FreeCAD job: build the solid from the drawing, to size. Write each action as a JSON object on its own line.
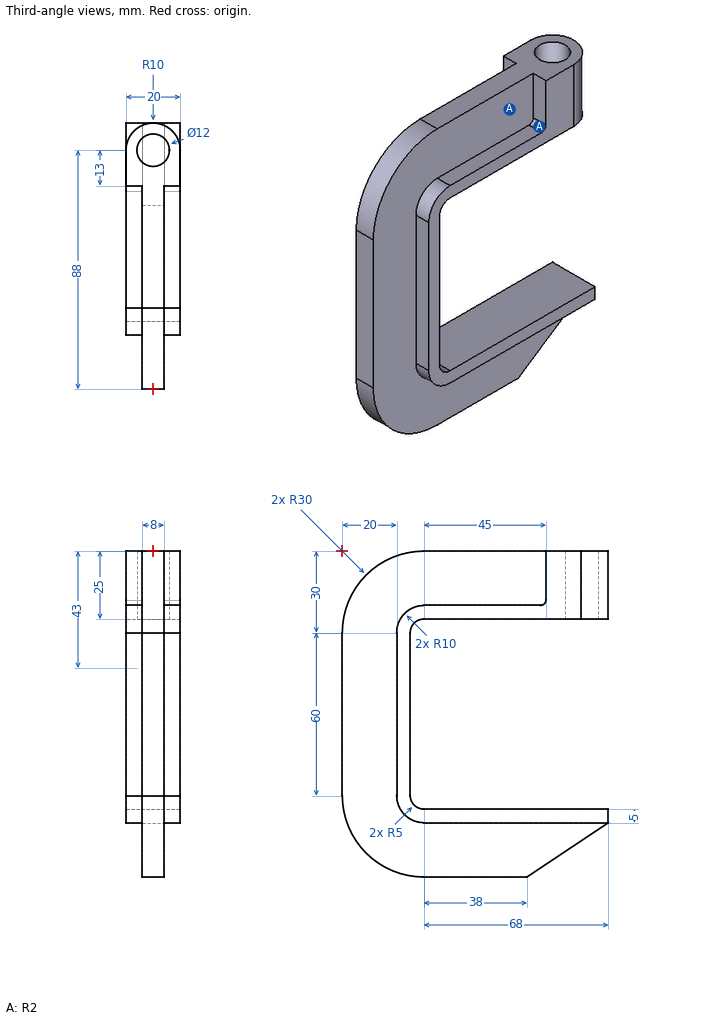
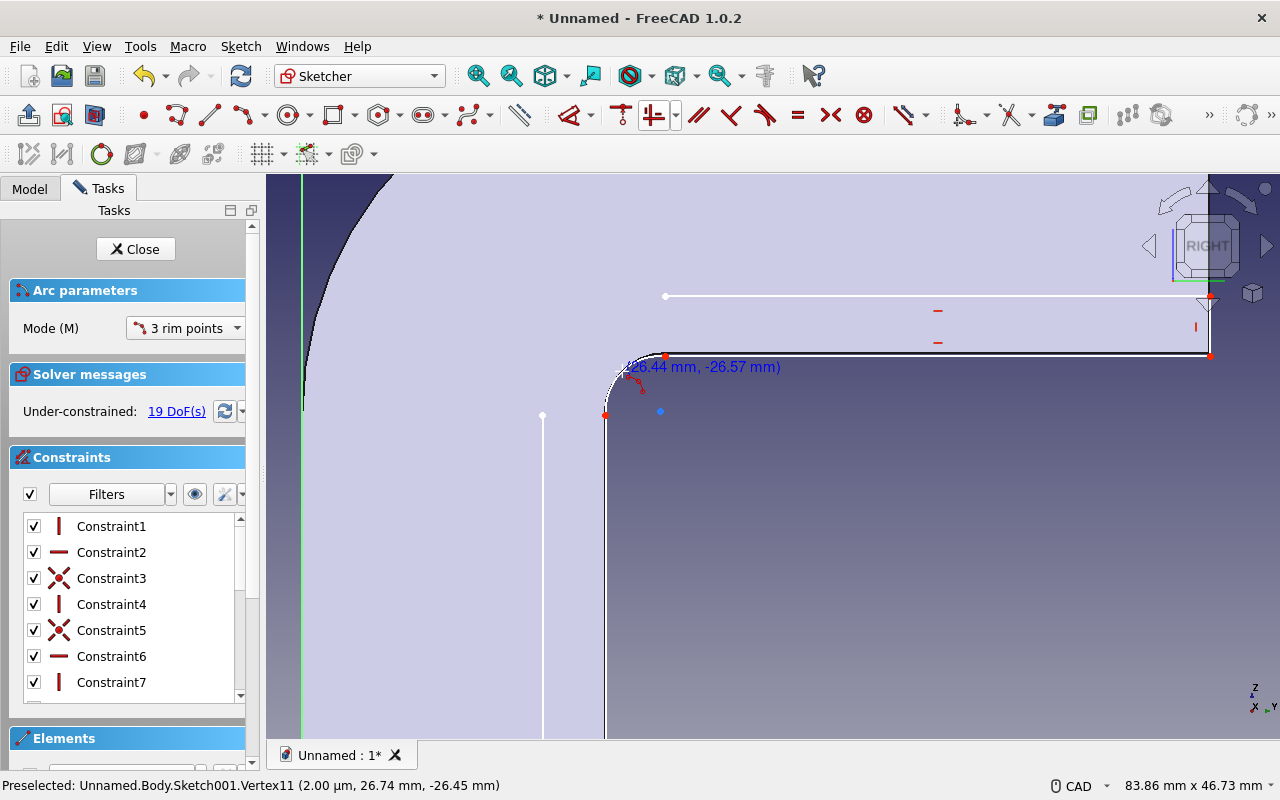
{"action": "left_click", "coordinate": [666, 296]}
{"action": "left_click", "coordinate": [543, 416]}
{"action": "left_click", "coordinate": [580, 328]}
{"action": "key", "text": "Escape"}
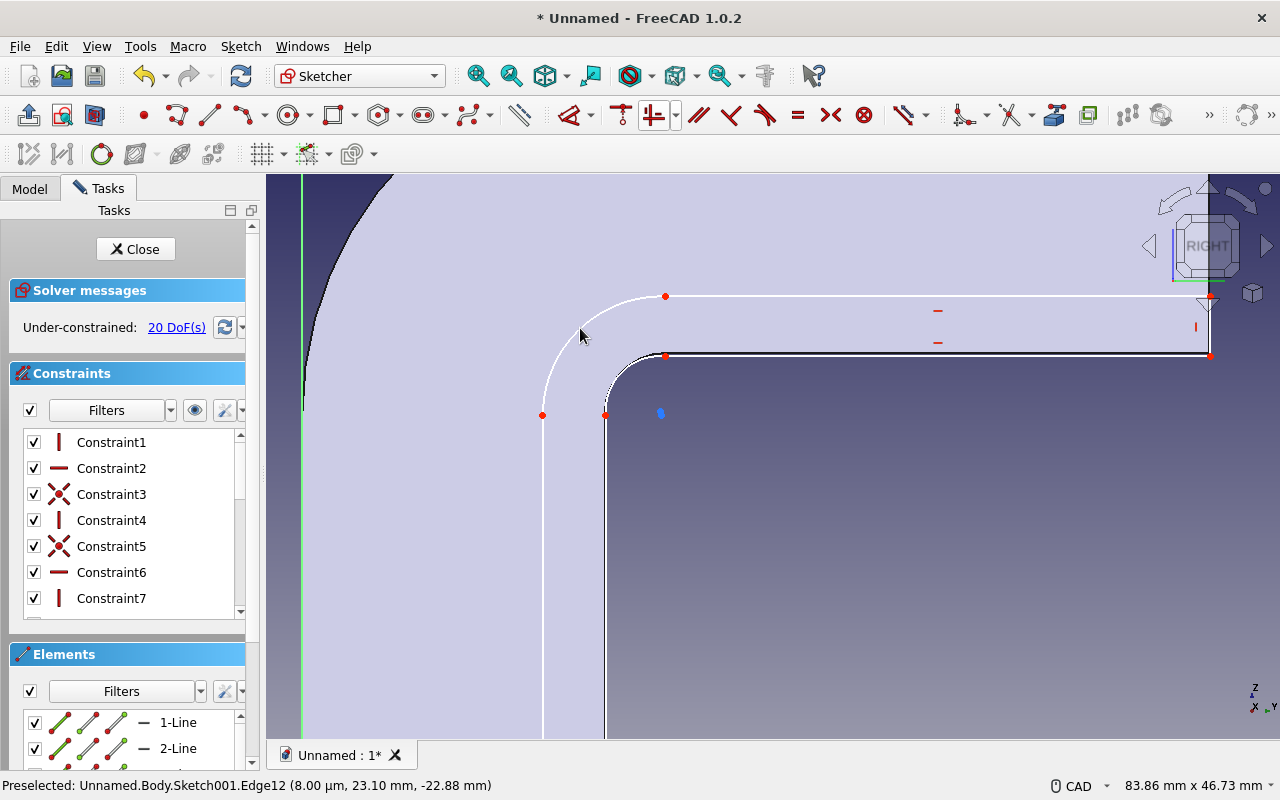
{"action": "left_click", "coordinate": [543, 634]}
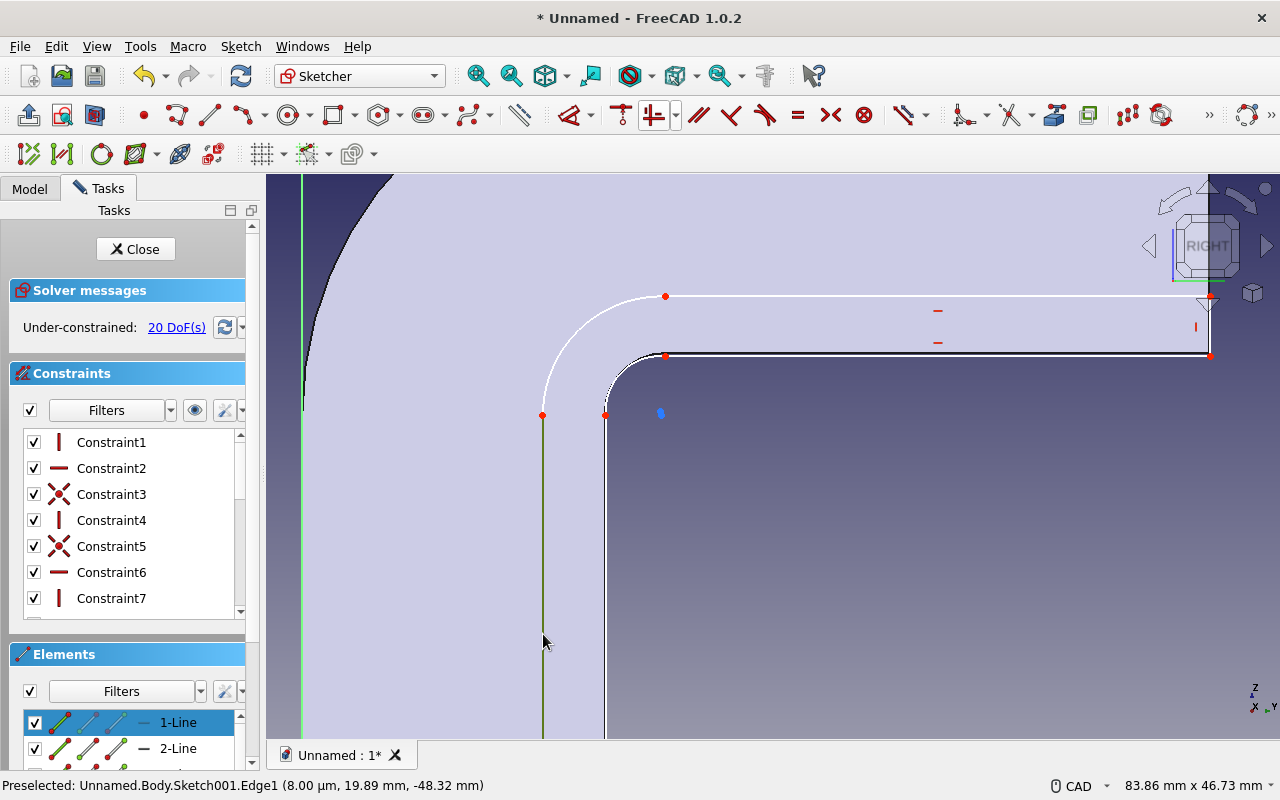
{"action": "scroll", "coordinate": [622, 371], "scroll_direction": "down", "scroll_amount": 6}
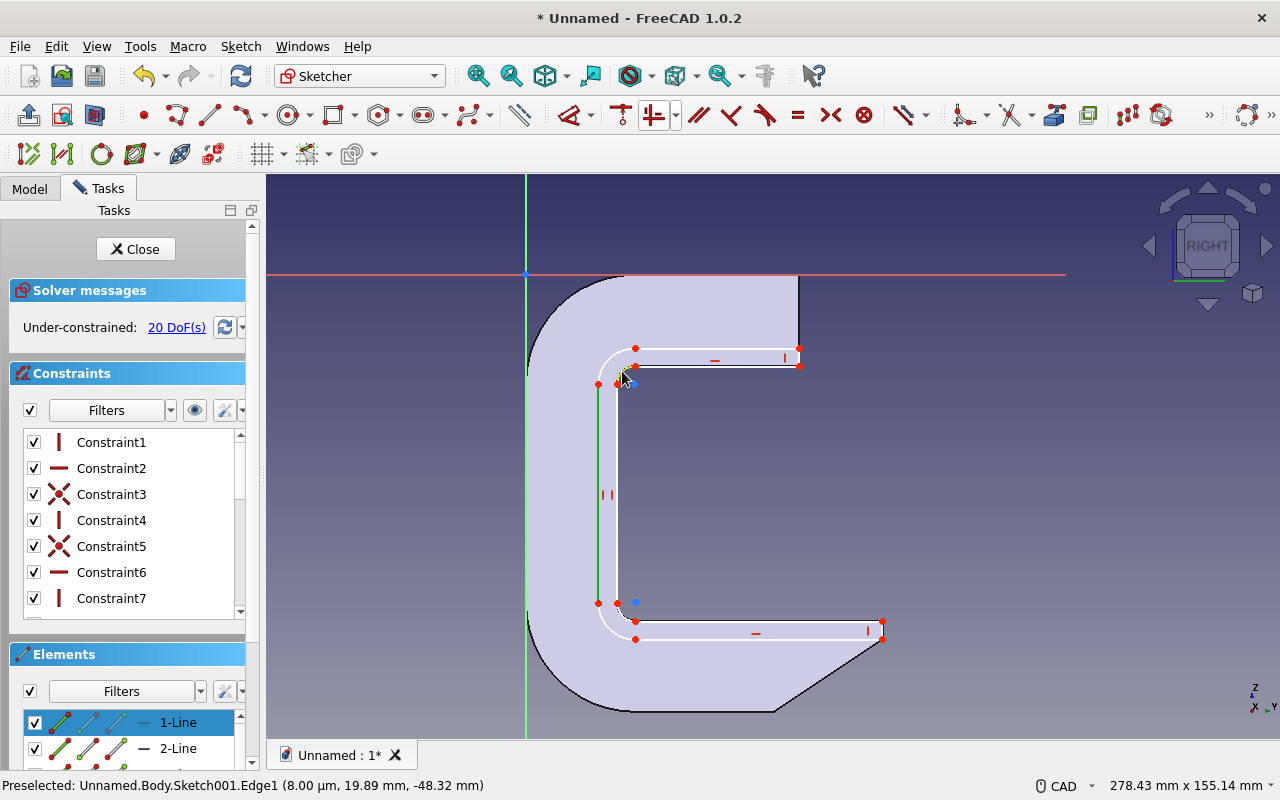
{"action": "left_click", "coordinate": [603, 620]}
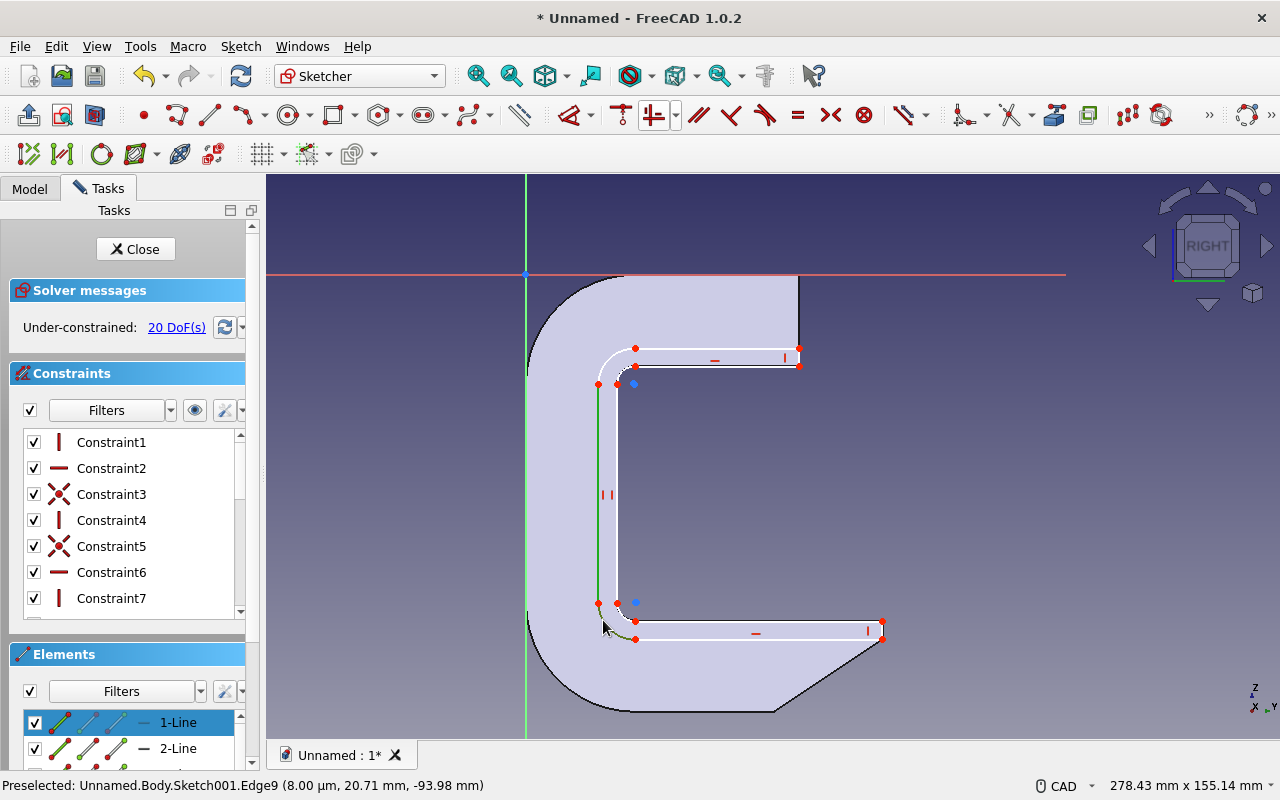
{"action": "left_click", "coordinate": [765, 116]}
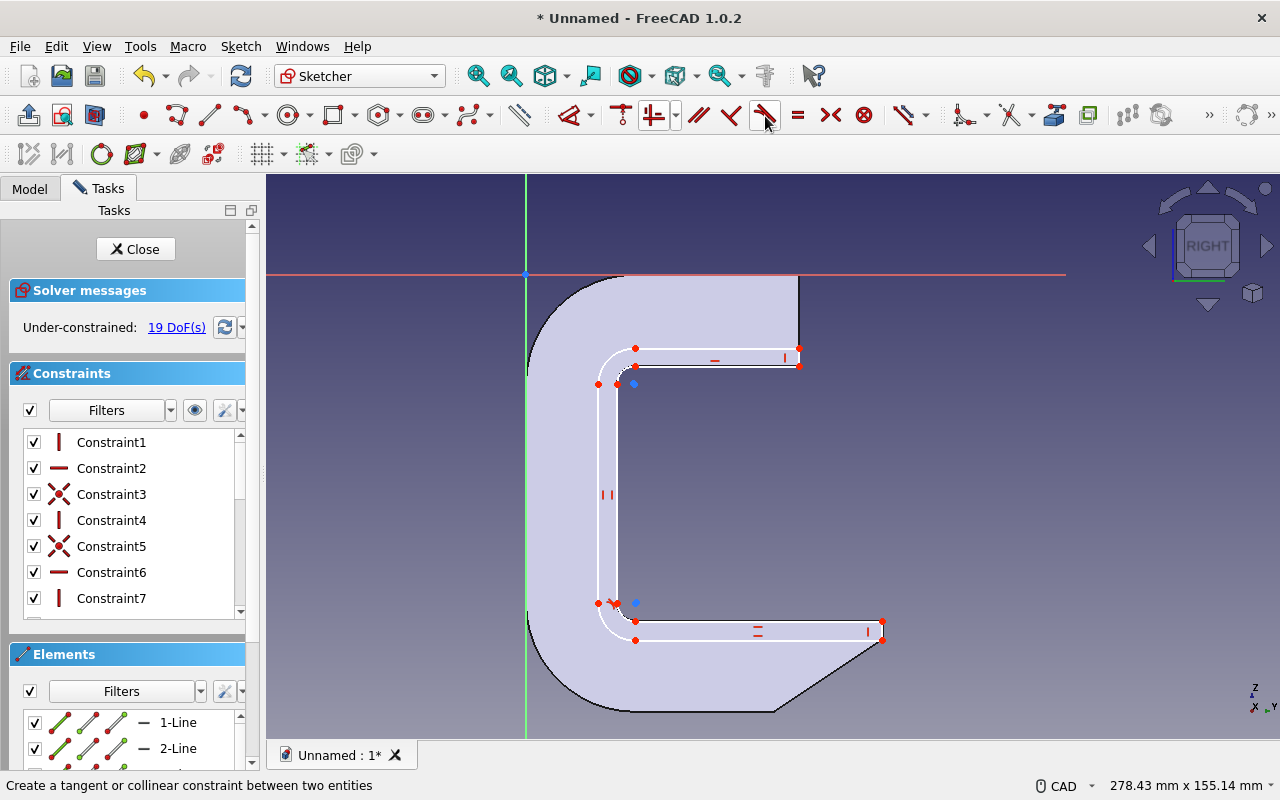
{"action": "left_click", "coordinate": [598, 450]}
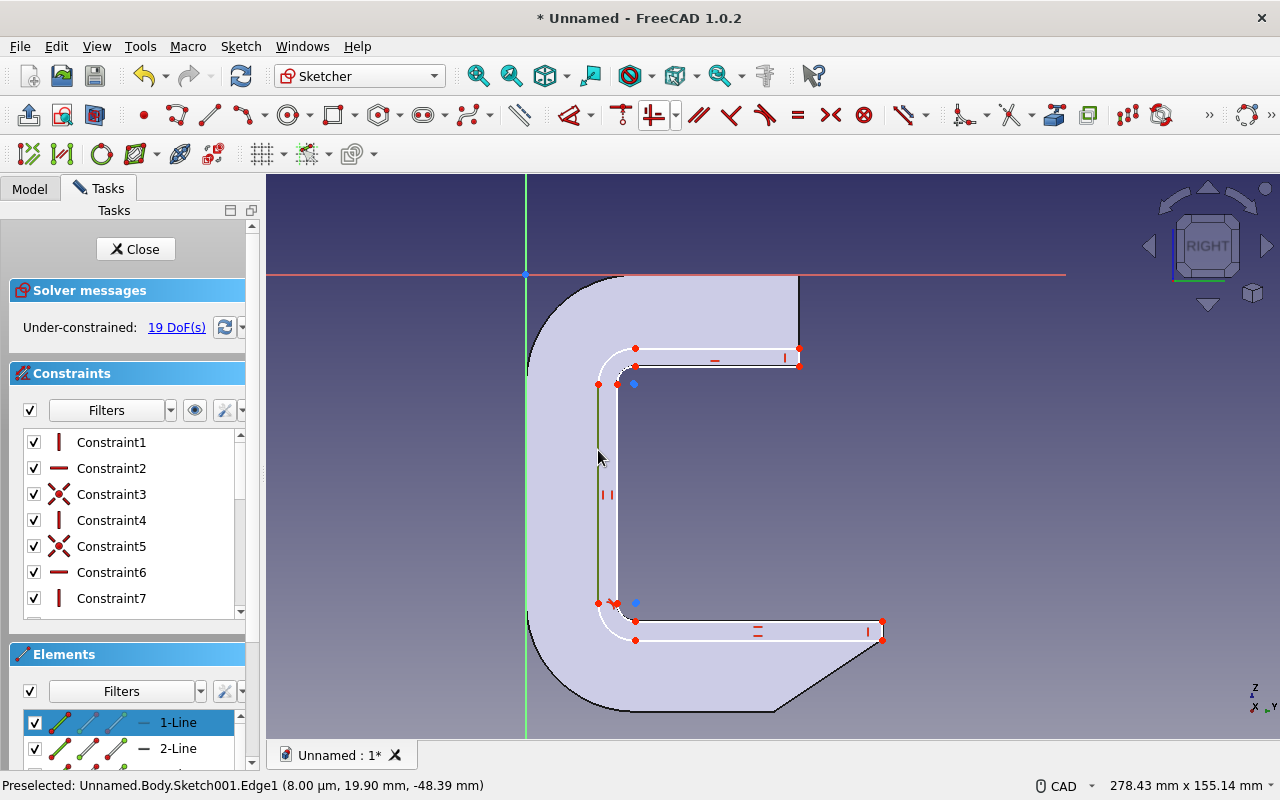
{"action": "left_click", "coordinate": [619, 352]}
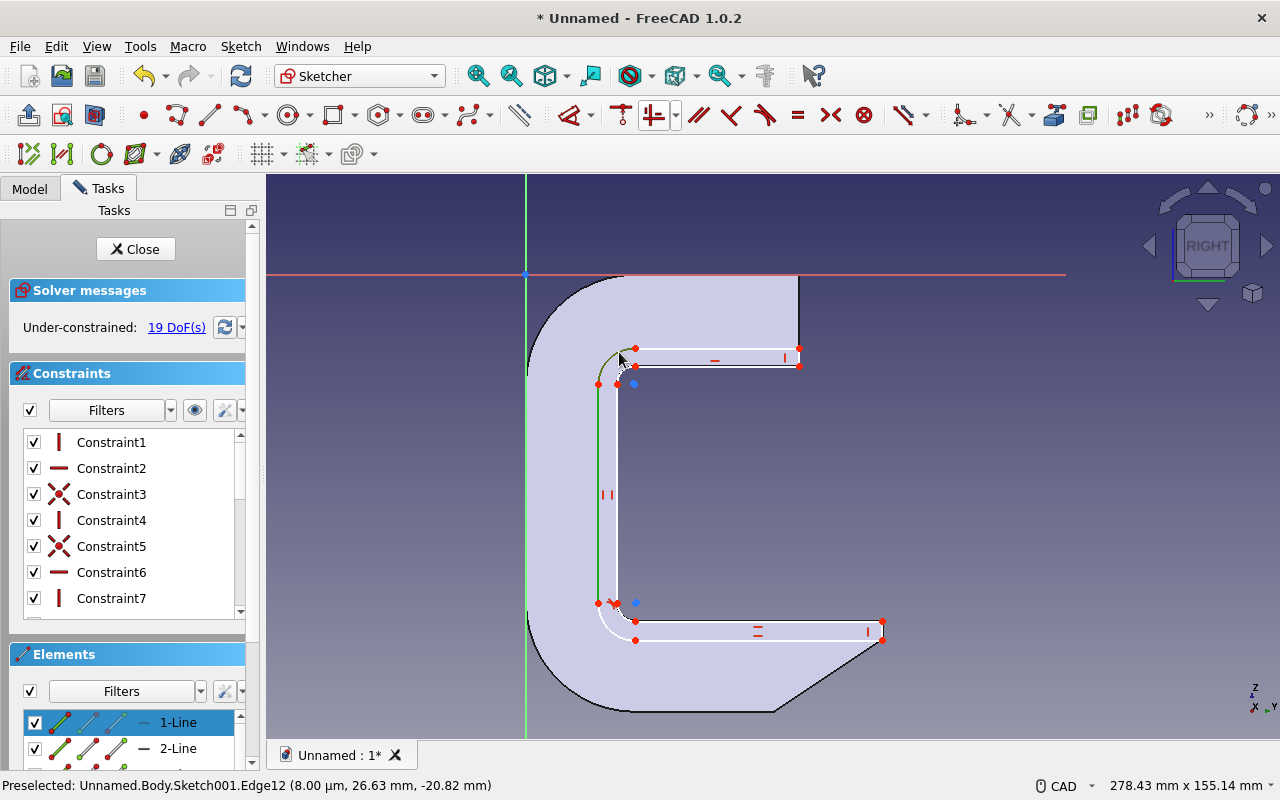
{"action": "key", "text": "t"}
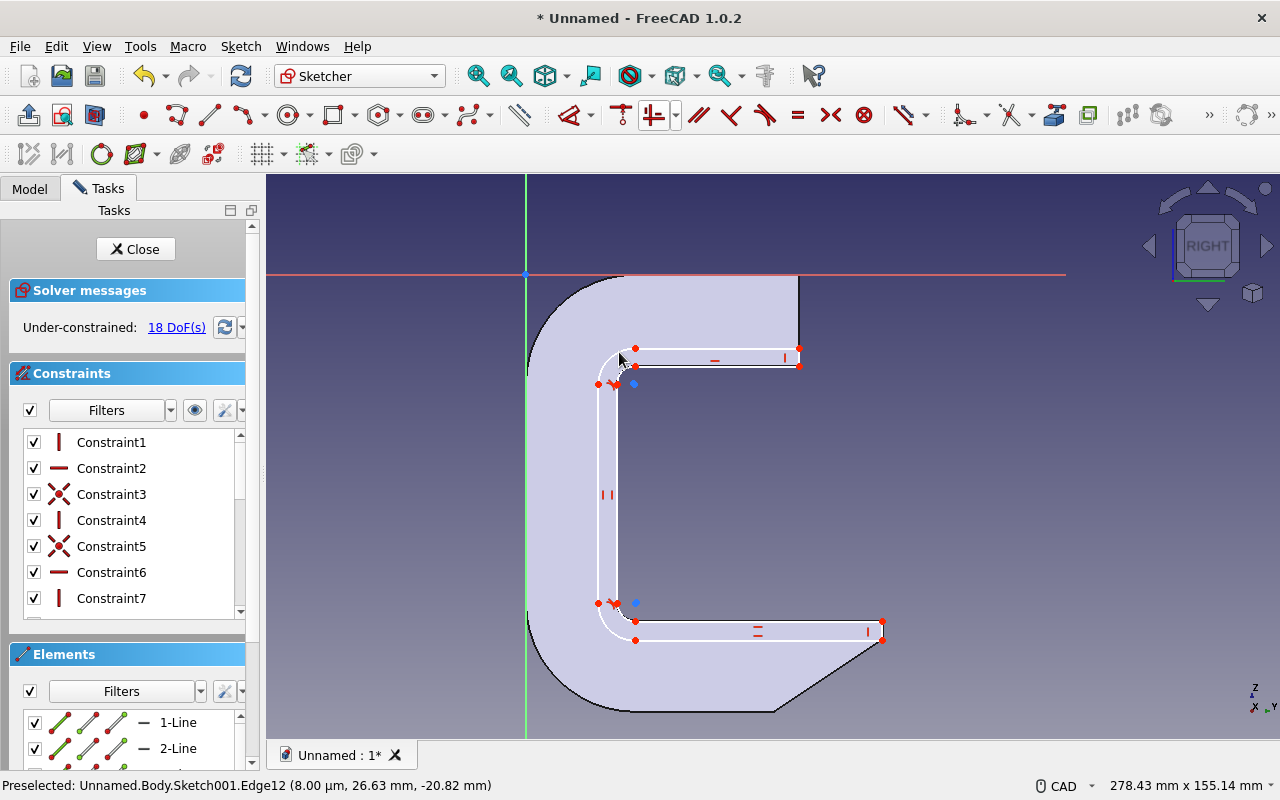
{"action": "left_click", "coordinate": [710, 641]}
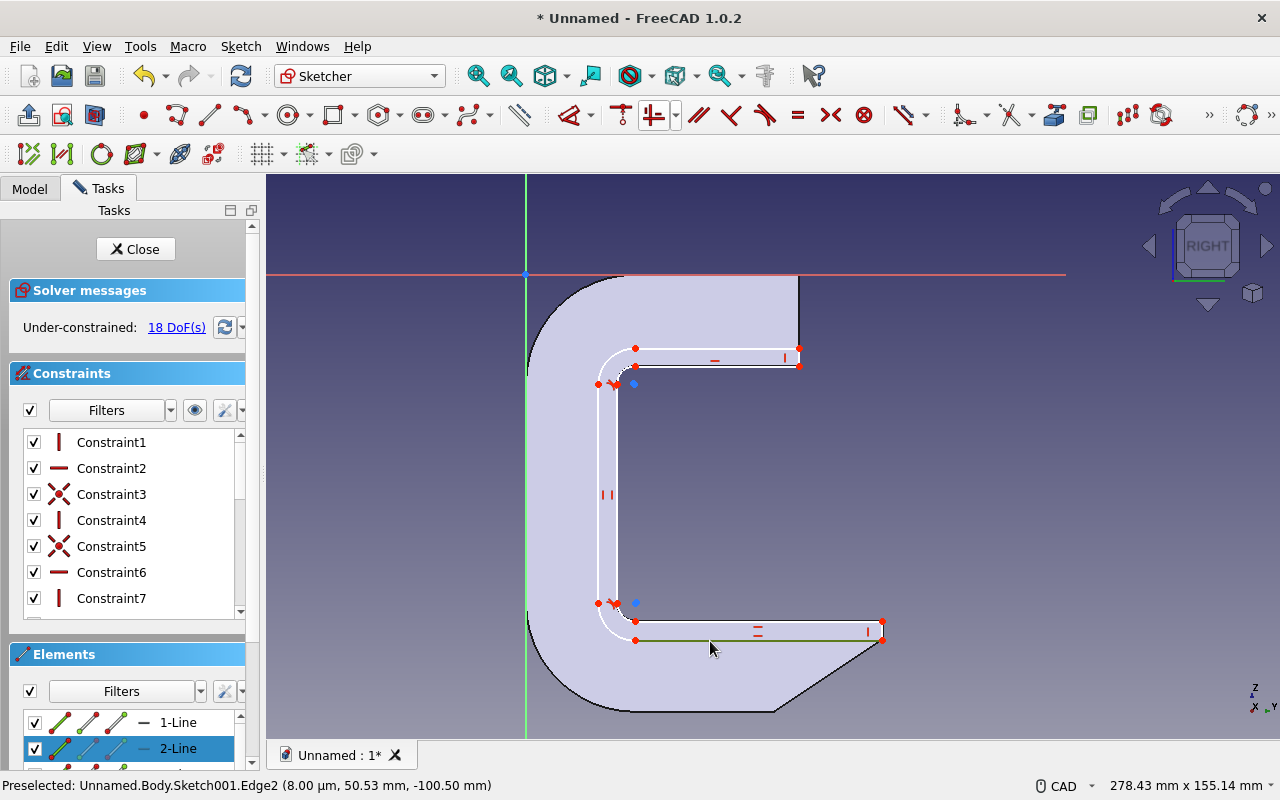
{"action": "left_click", "coordinate": [602, 620]}